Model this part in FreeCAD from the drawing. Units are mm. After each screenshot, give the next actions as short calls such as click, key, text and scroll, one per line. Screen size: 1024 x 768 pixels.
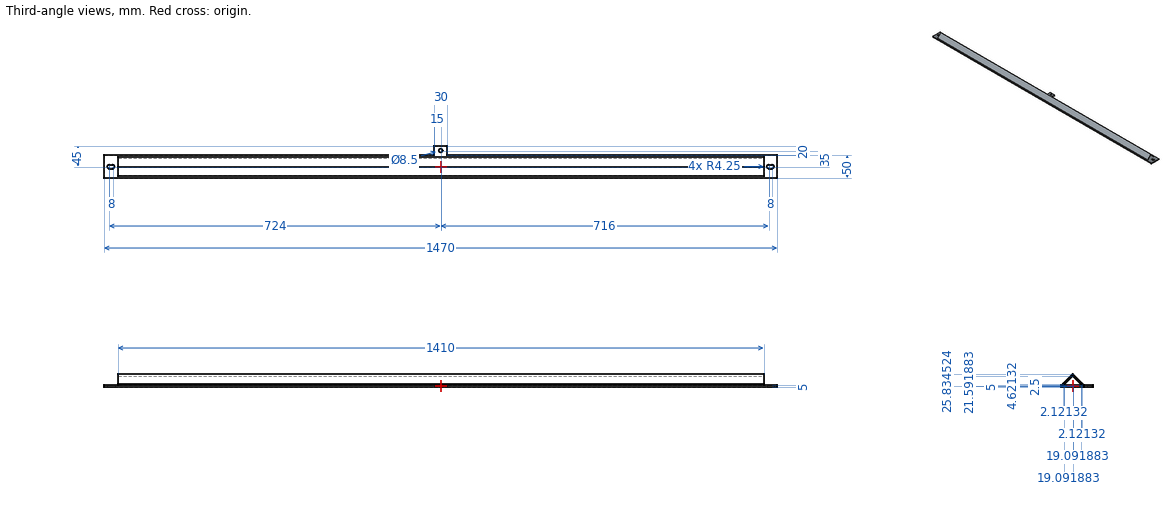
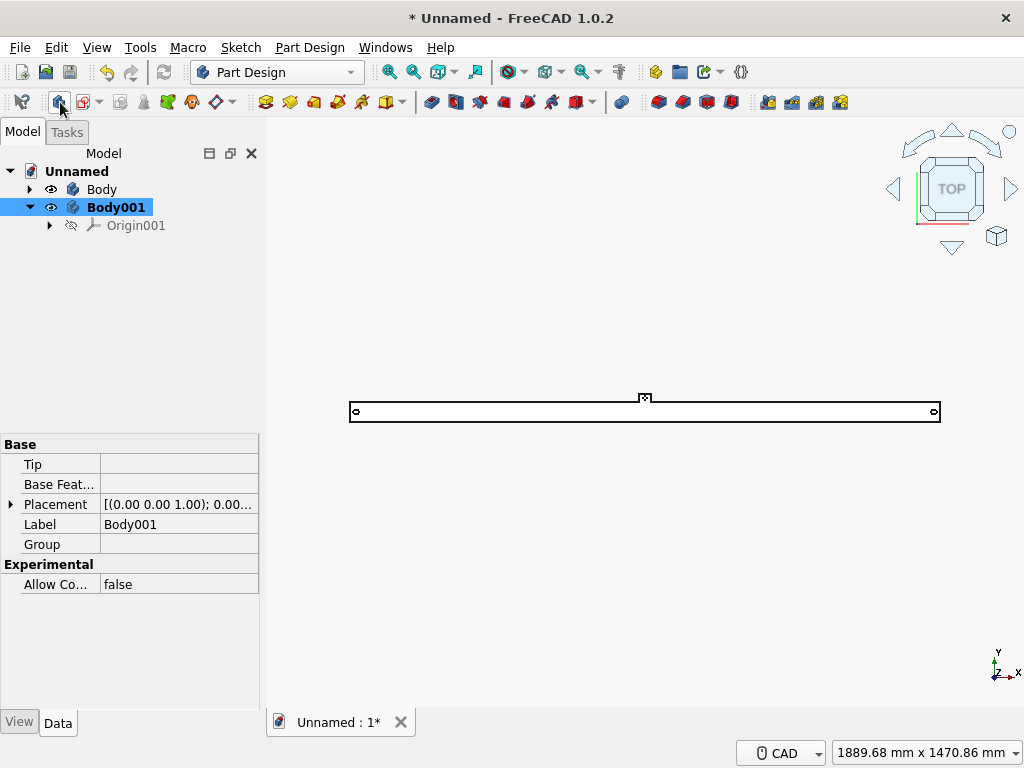
click(50, 225)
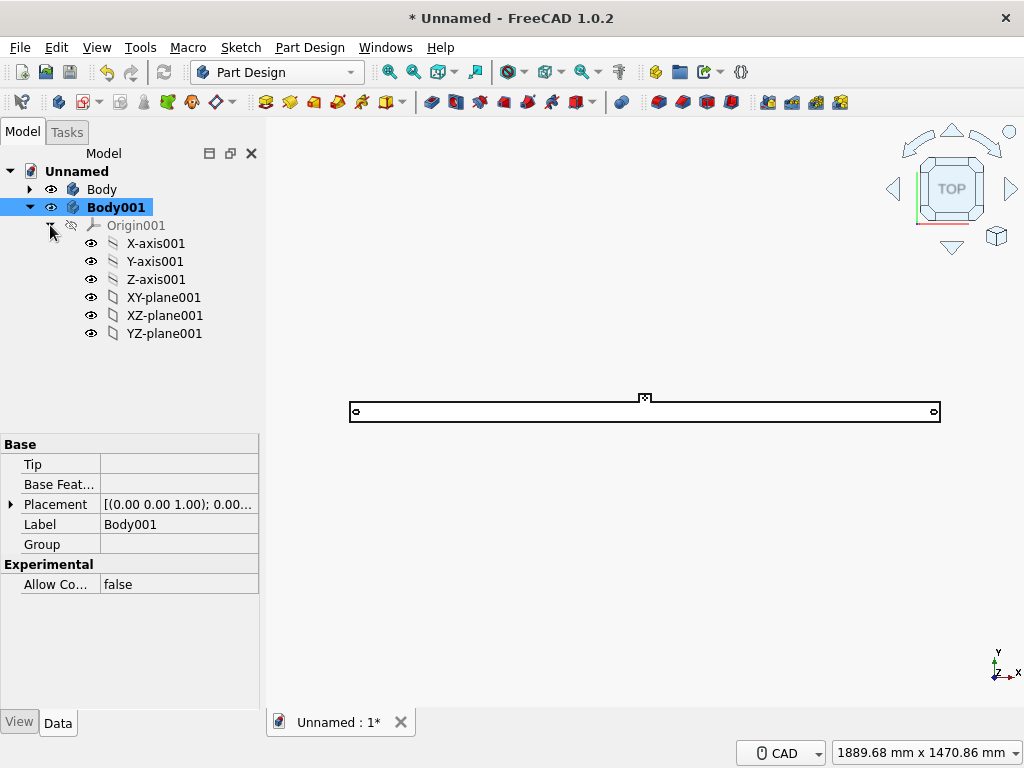
click(136, 333)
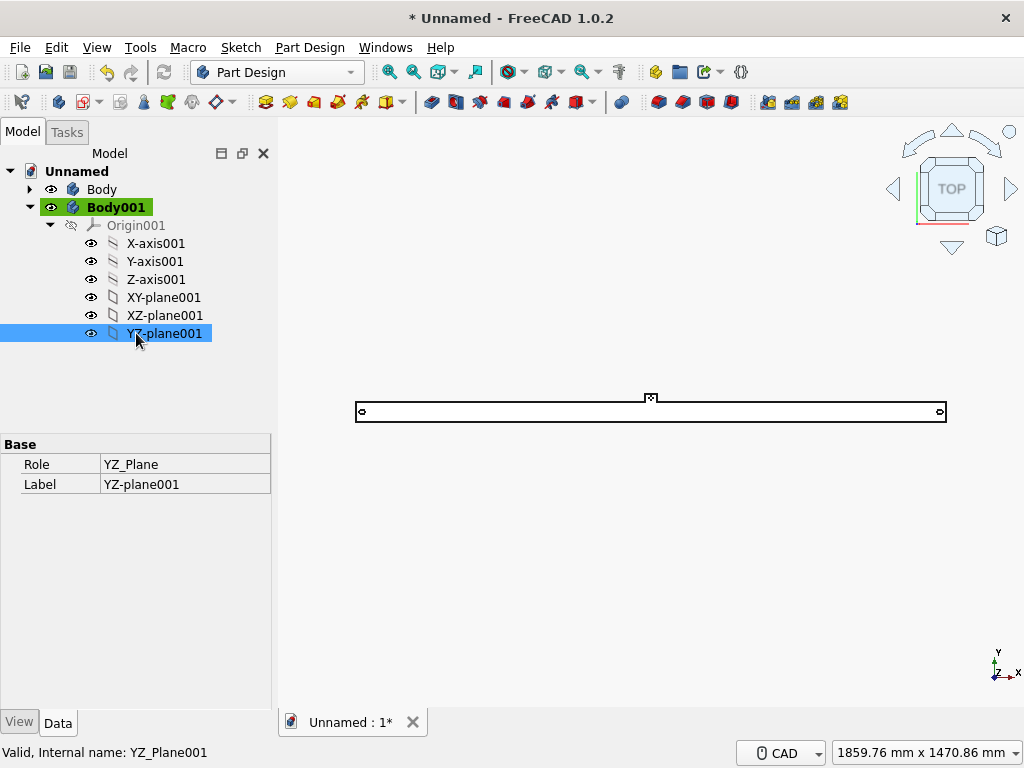
click(216, 102)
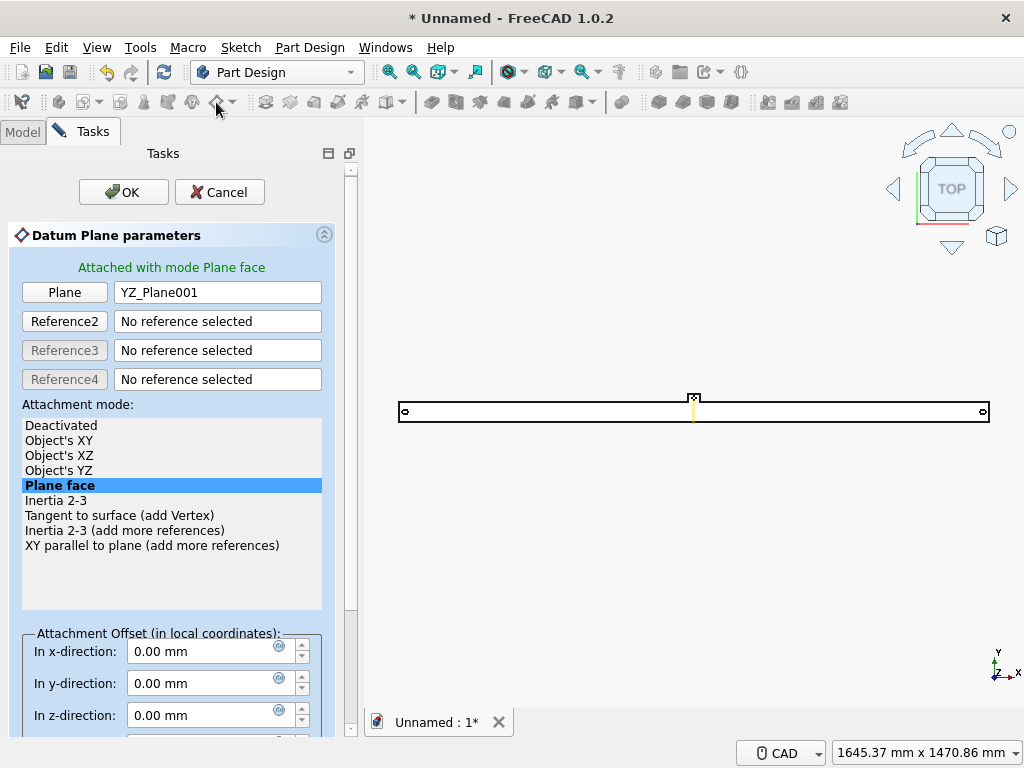
triple_click(210, 715)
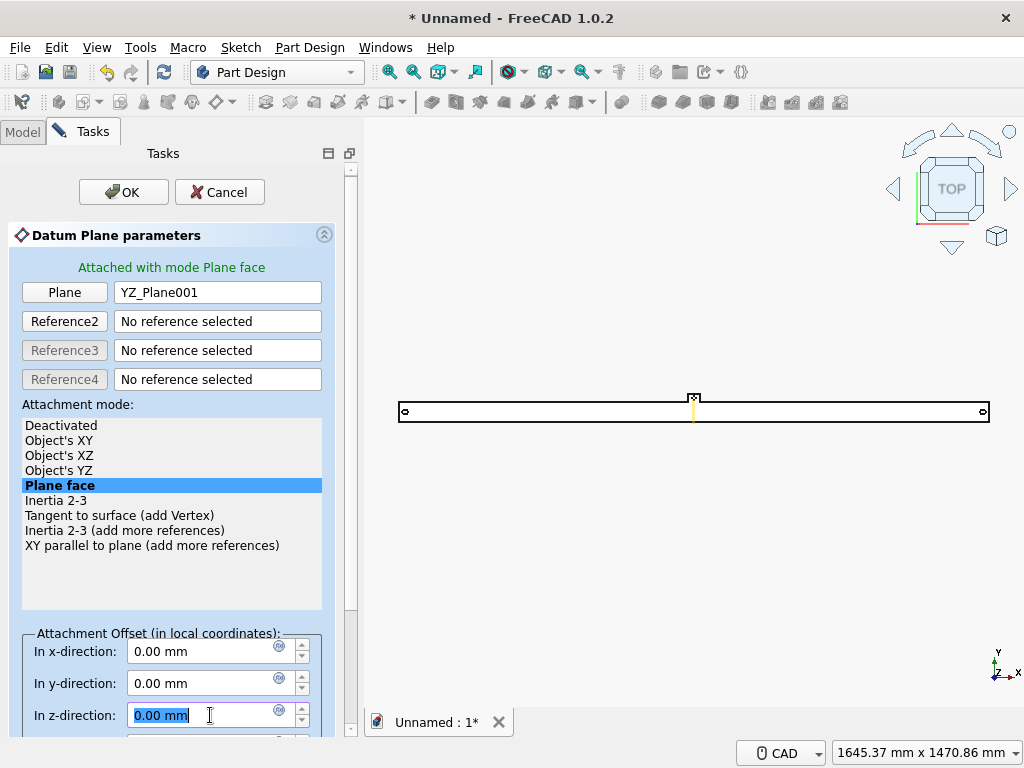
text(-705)
key(Tab)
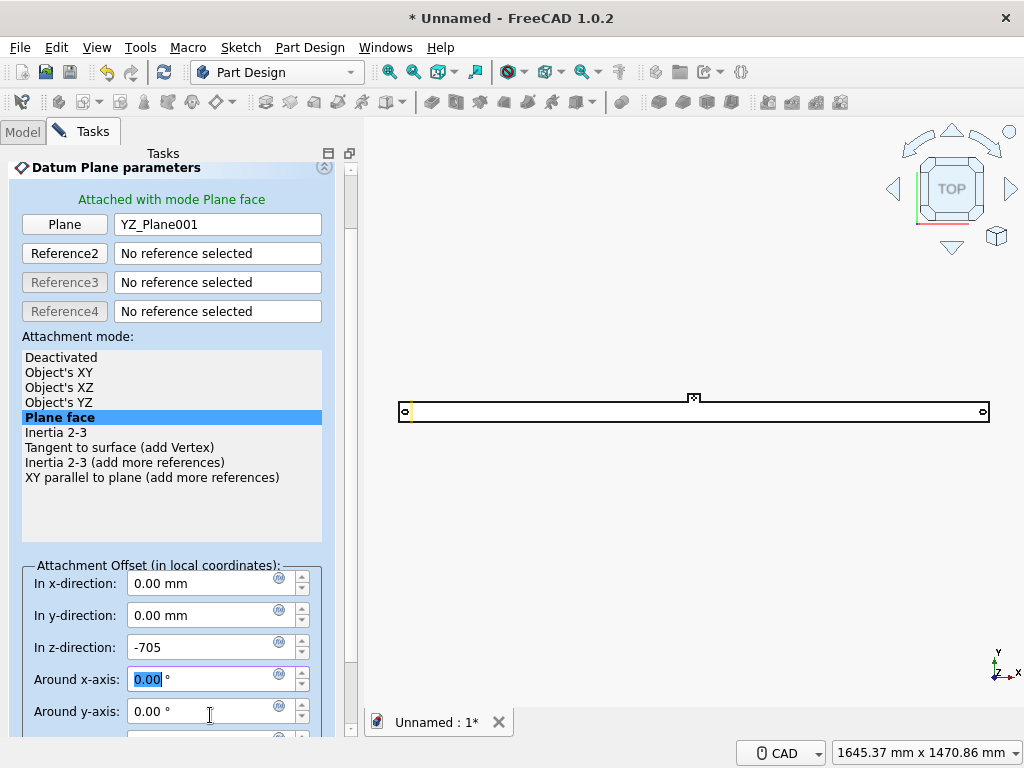
scroll(351, 450, up, 2)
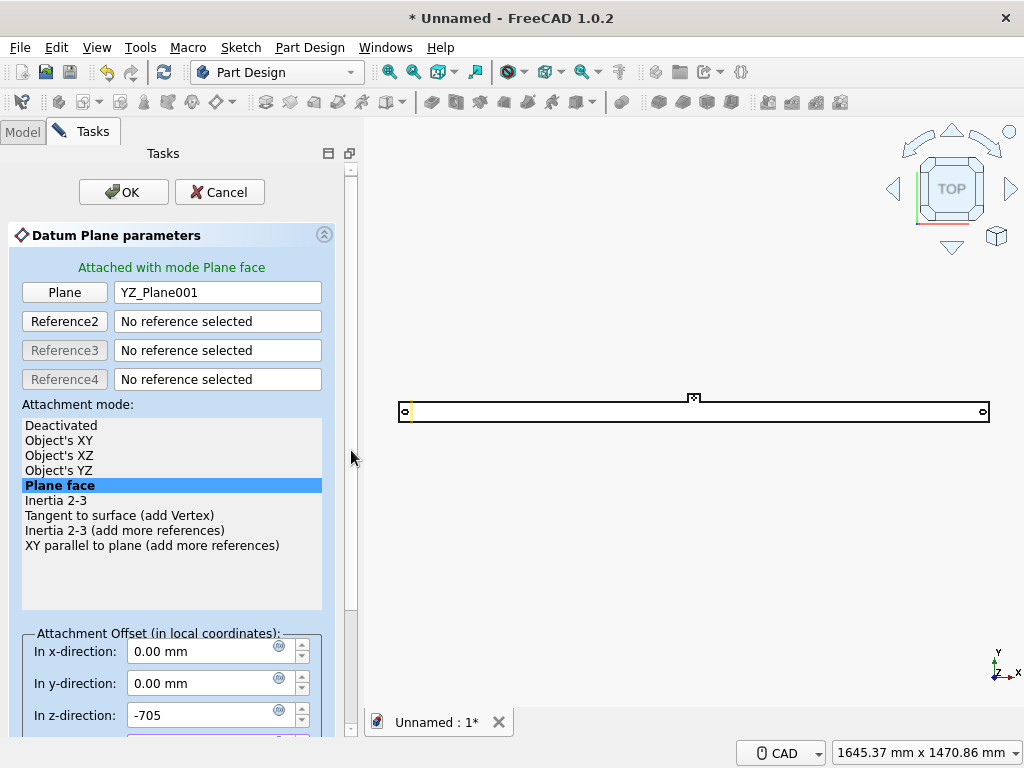
click(124, 192)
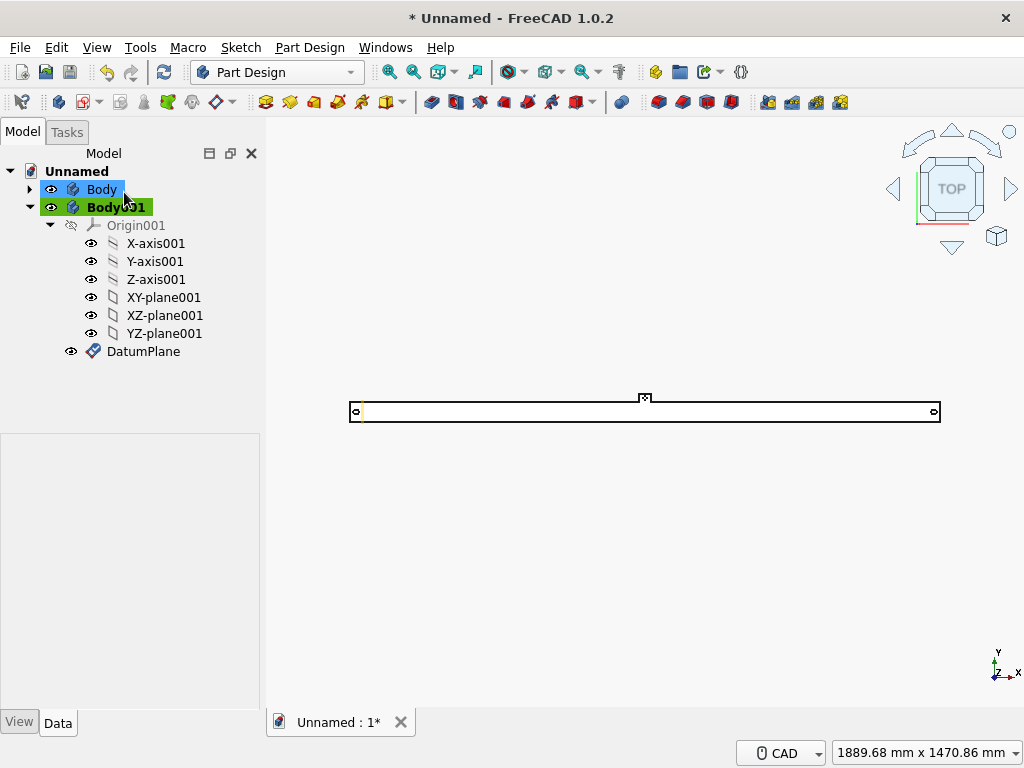
click(116, 351)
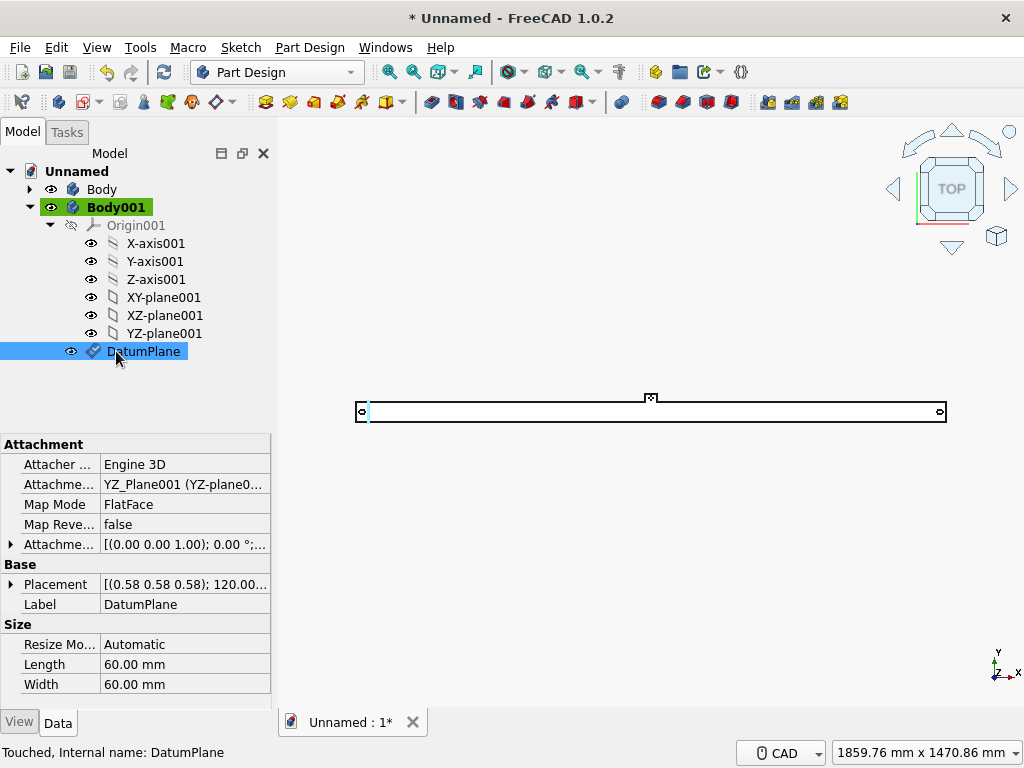
click(84, 102)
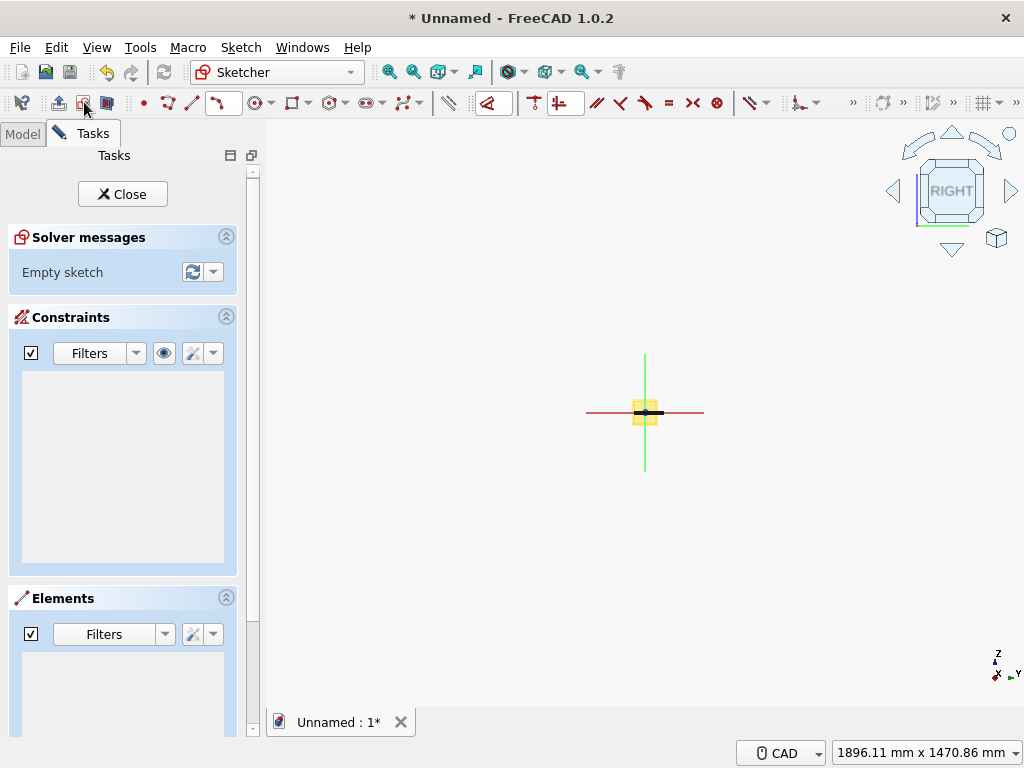
scroll(649, 408, up, 15)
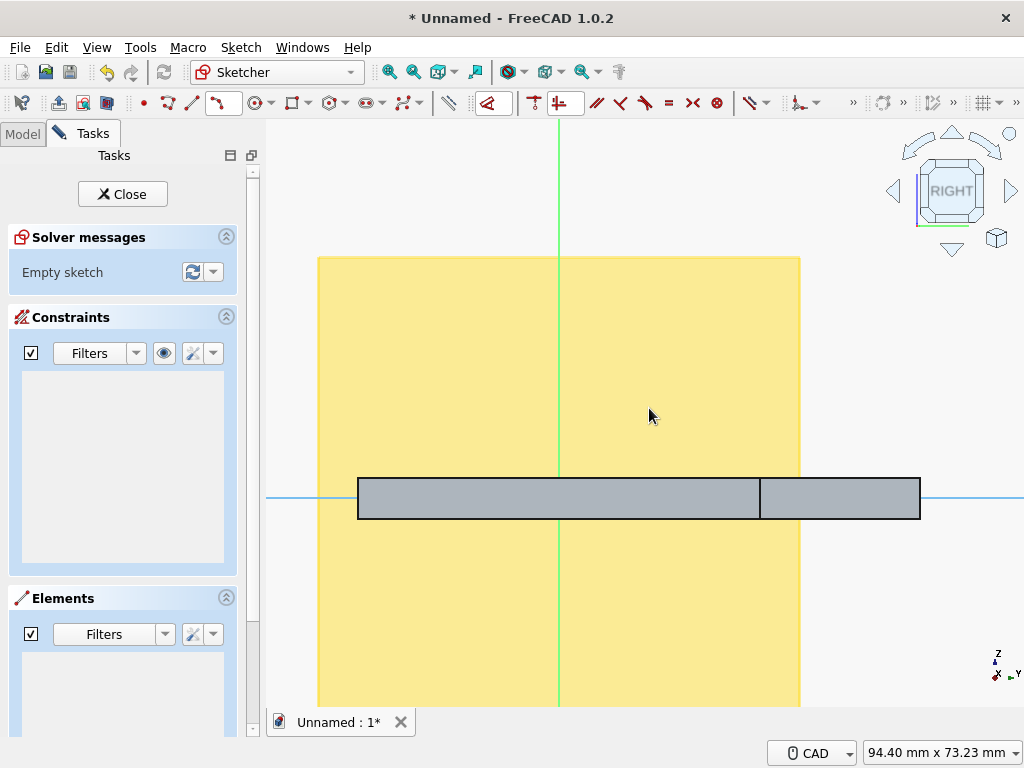
key(g)
key(m)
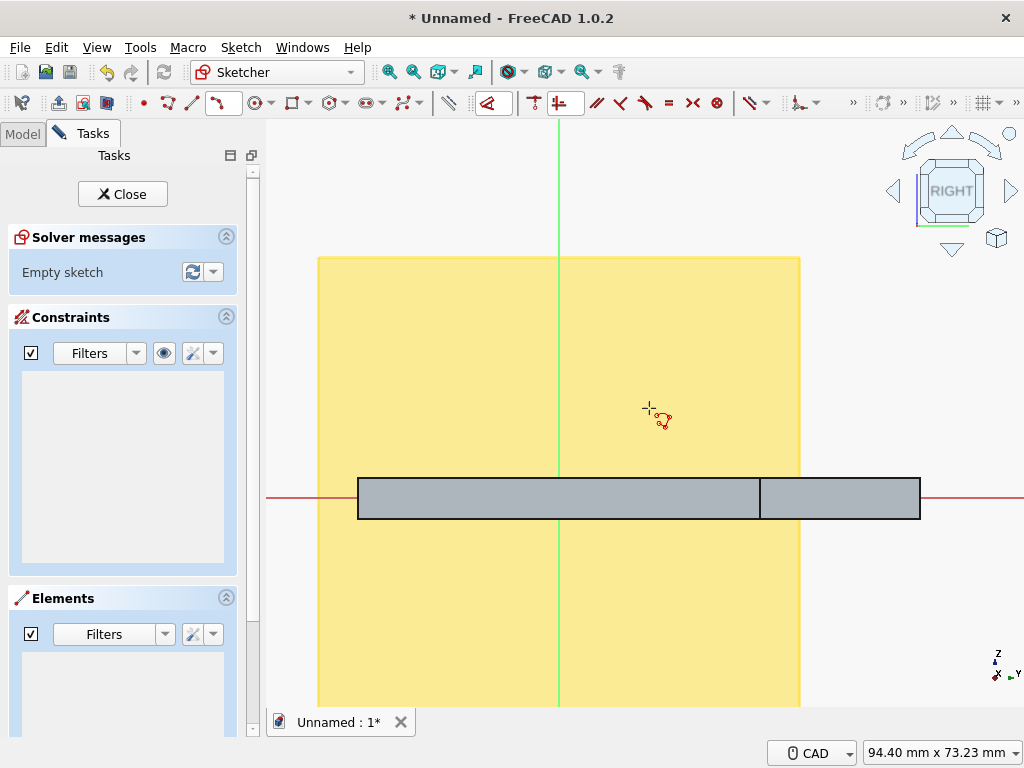
click(712, 478)
click(559, 325)
click(406, 478)
click(389, 461)
click(559, 291)
click(729, 461)
click(712, 479)
key(Escape)
key(Escape)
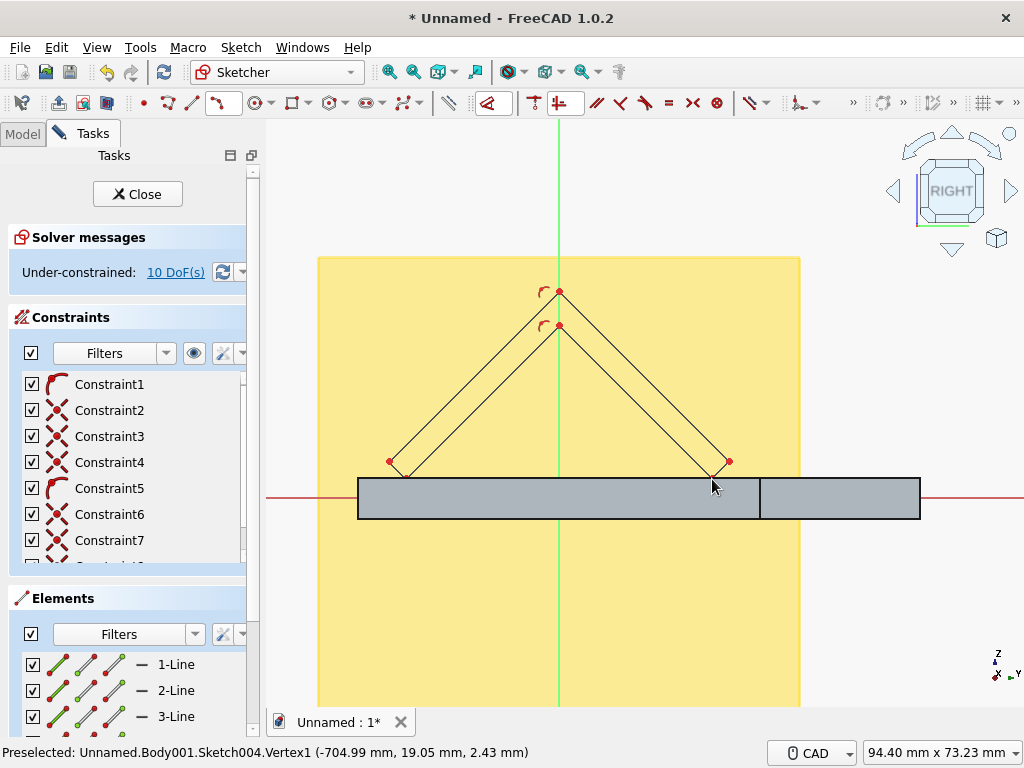
scroll(712, 479, up, 4)